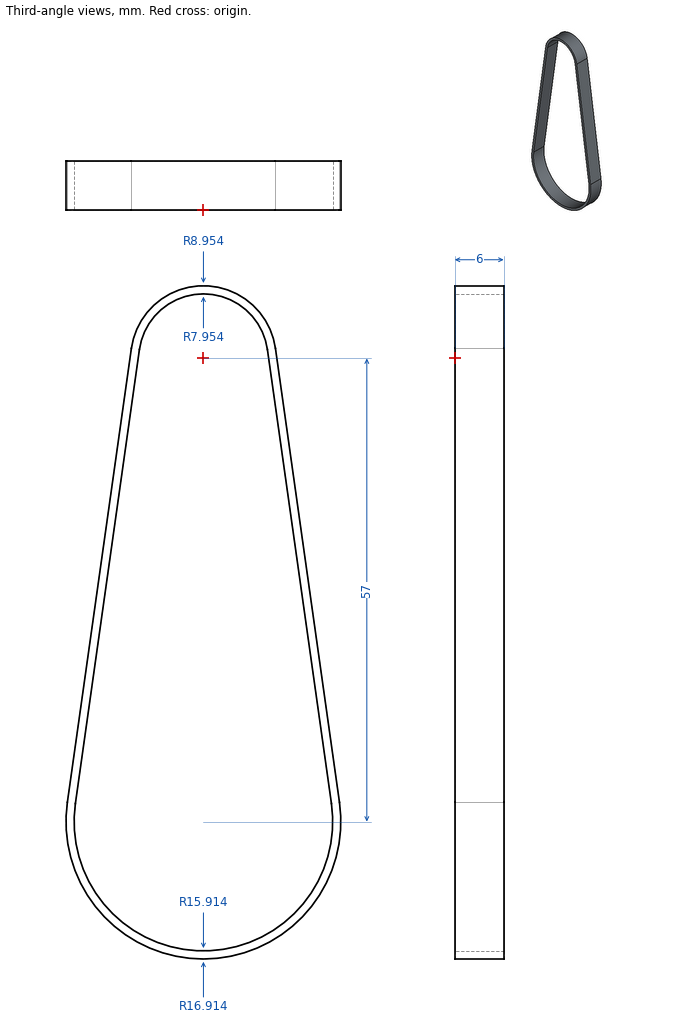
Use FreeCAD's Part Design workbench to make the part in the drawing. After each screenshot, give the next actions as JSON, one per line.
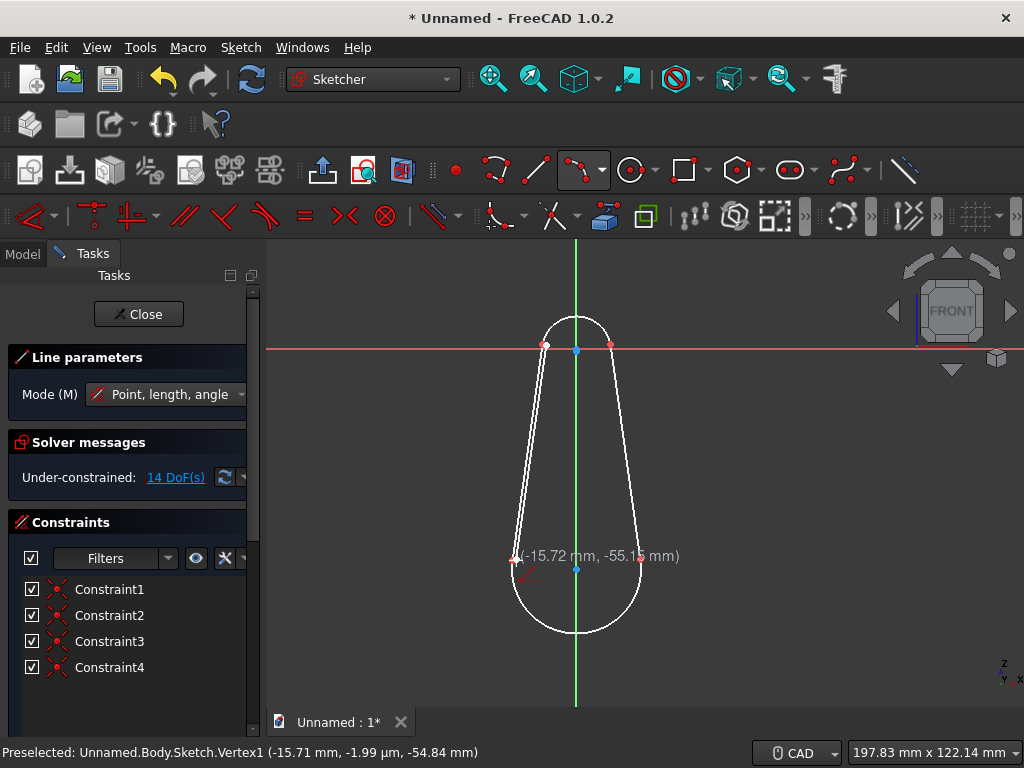
{"action": "scroll", "coordinate": [637, 559], "scroll_direction": "up", "scroll_amount": 8}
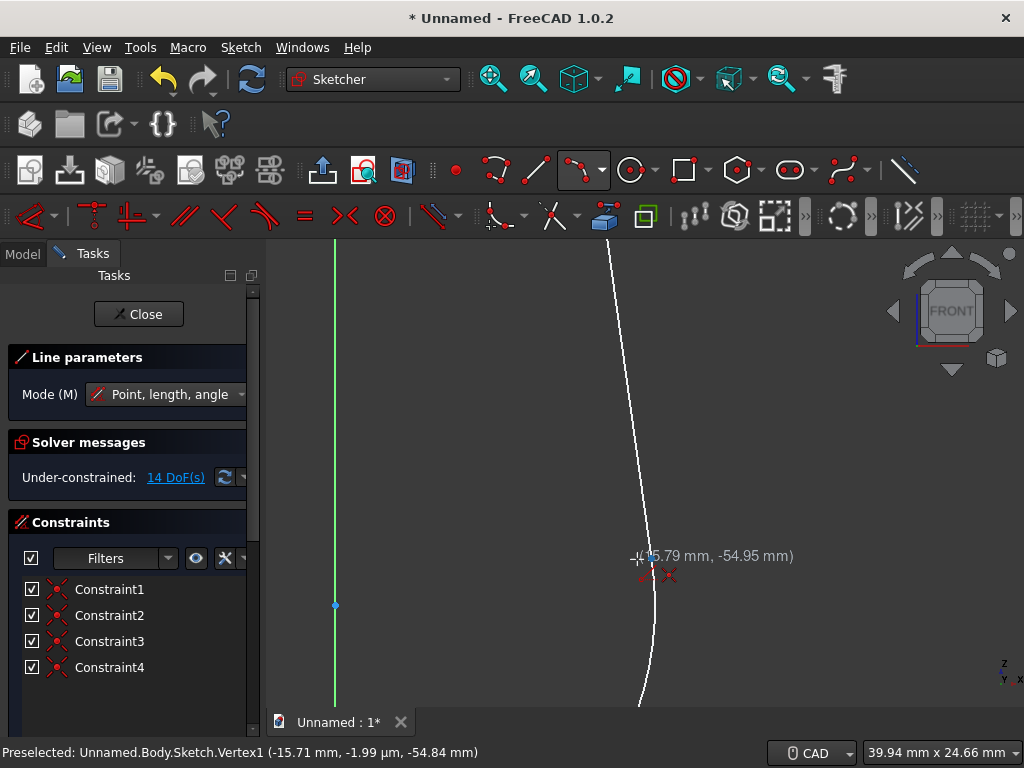
{"action": "left_click", "coordinate": [634, 558]}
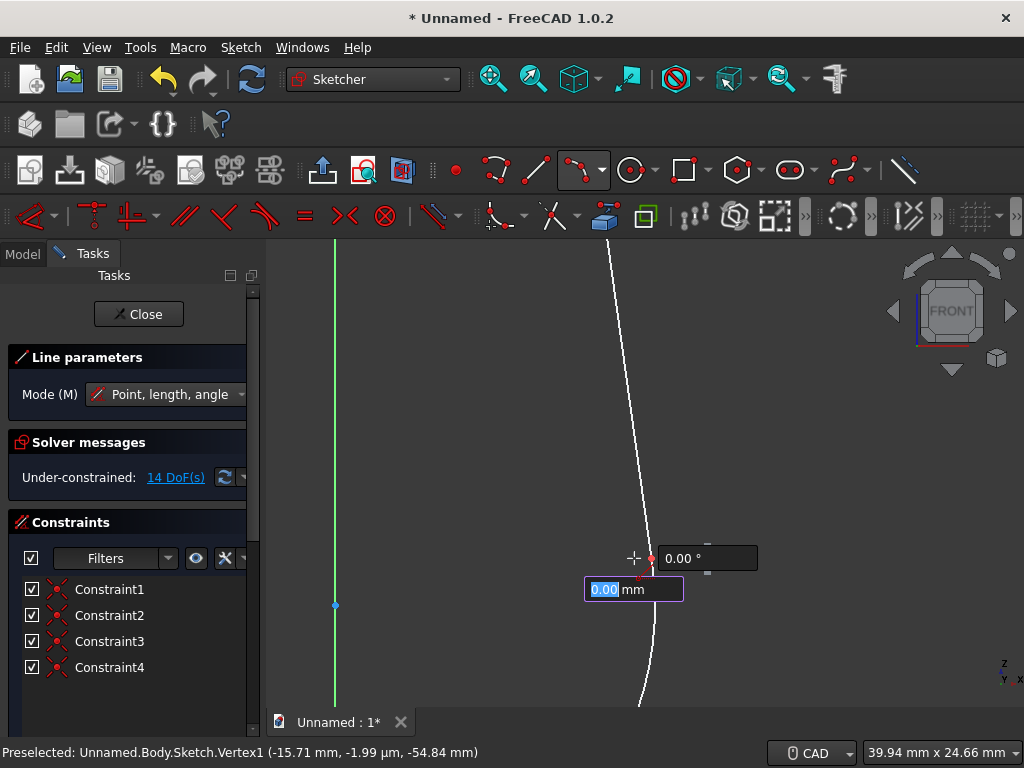
{"action": "scroll", "coordinate": [637, 559], "scroll_direction": "down", "scroll_amount": 8}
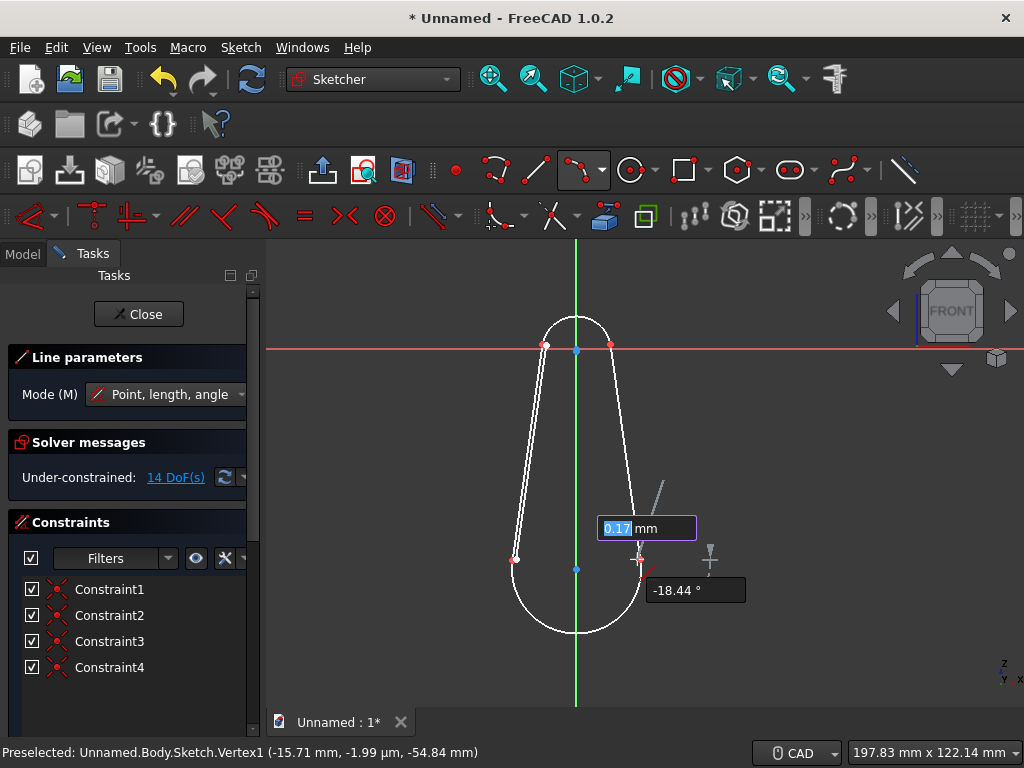
{"action": "scroll", "coordinate": [607, 345], "scroll_direction": "up", "scroll_amount": 8}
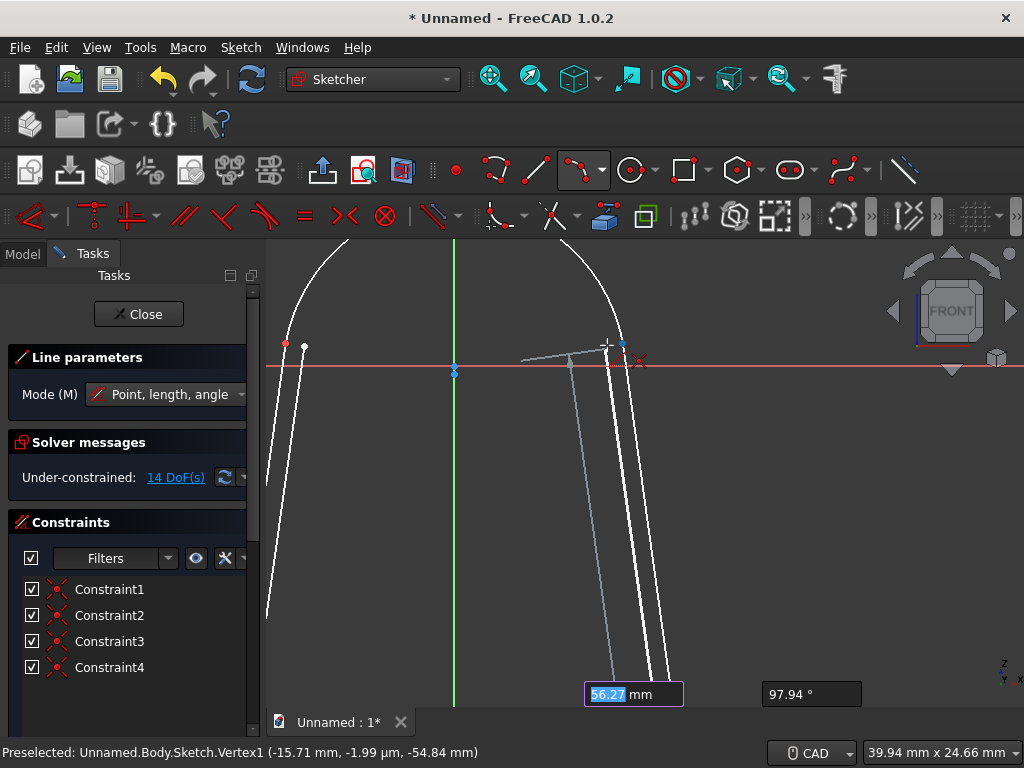
{"action": "left_click", "coordinate": [604, 345]}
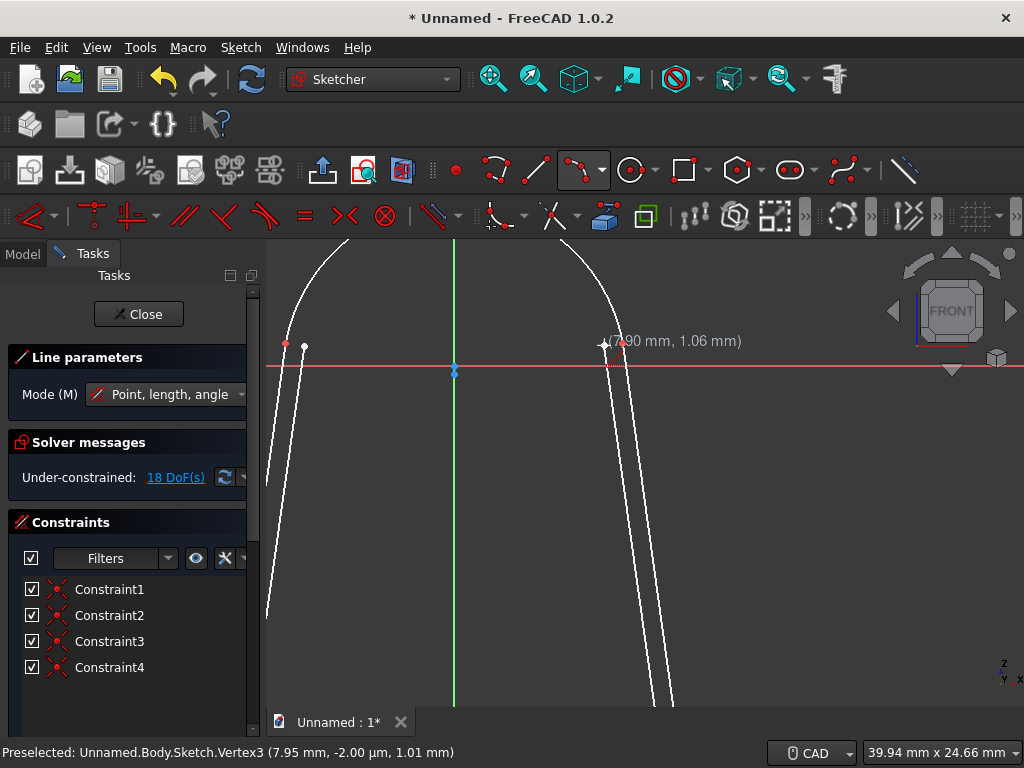
{"action": "left_click", "coordinate": [578, 170]}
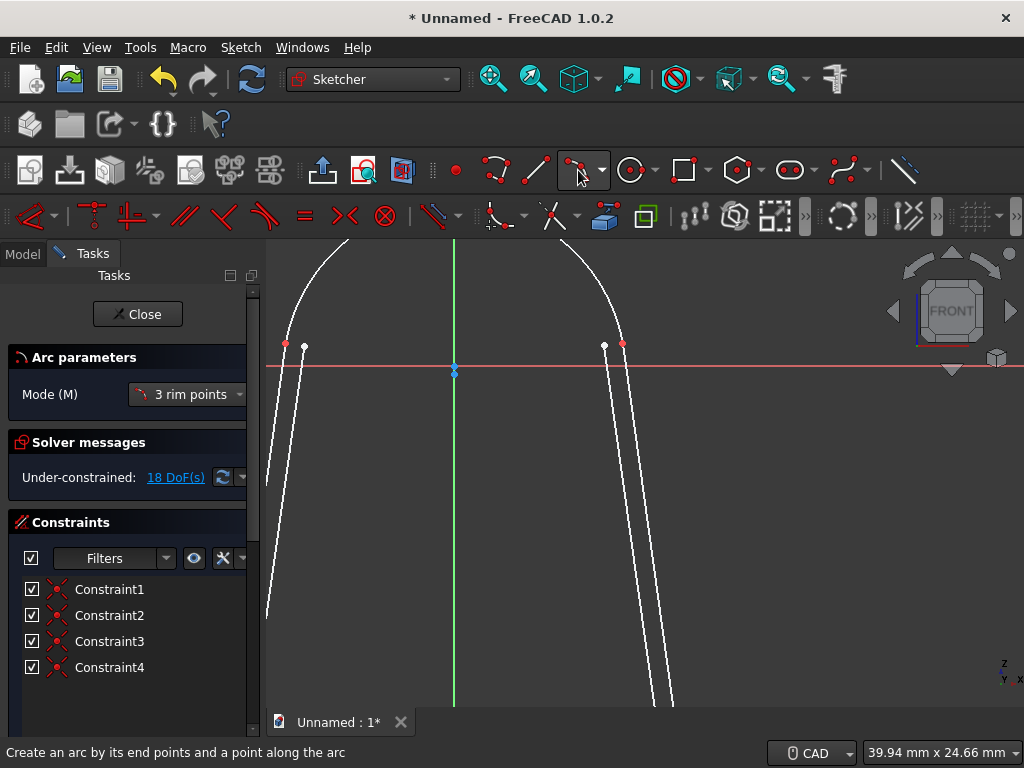
{"action": "scroll", "coordinate": [607, 344], "scroll_direction": "down", "scroll_amount": 8}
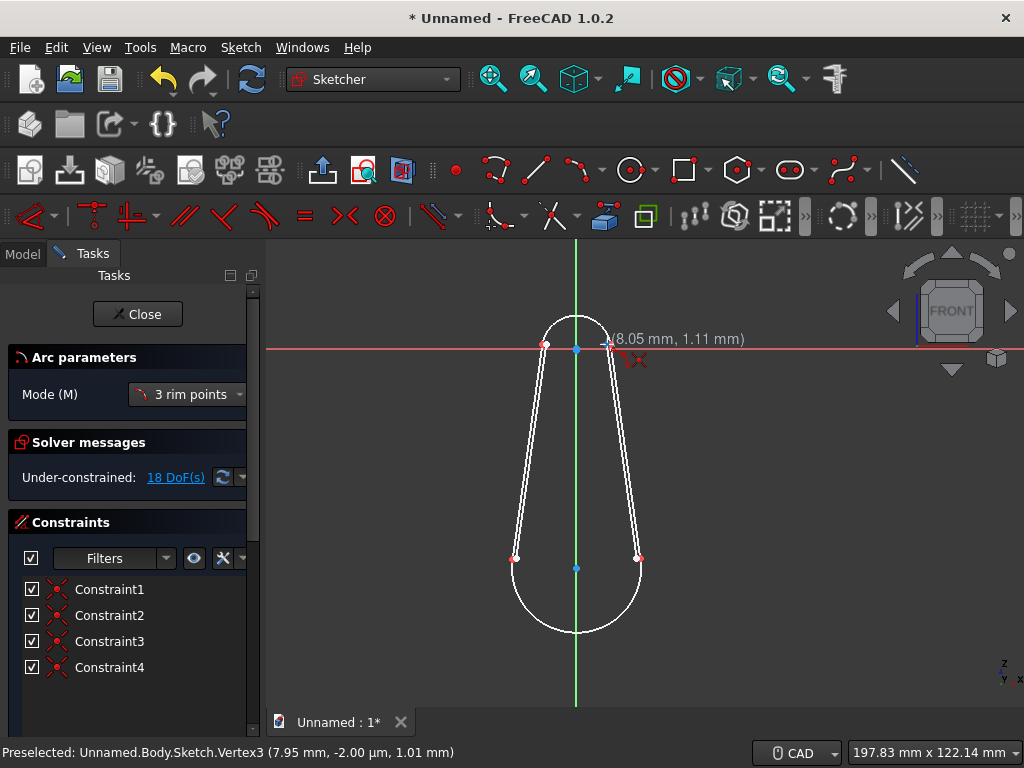
{"action": "scroll", "coordinate": [516, 559], "scroll_direction": "up", "scroll_amount": 8}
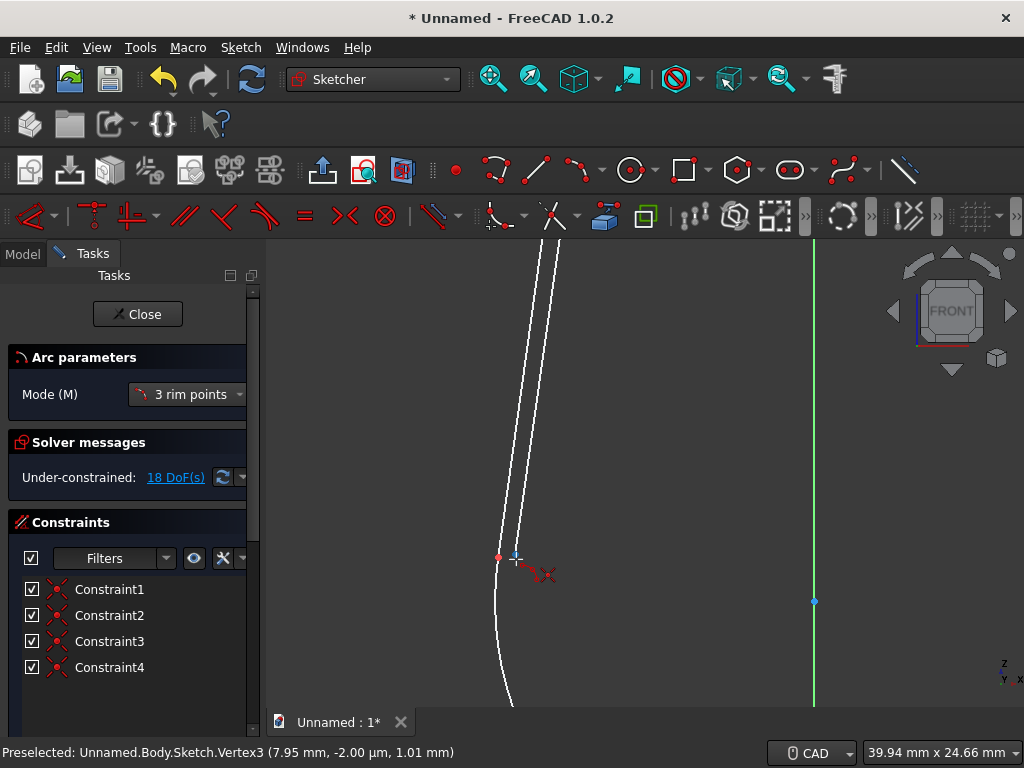
{"action": "left_click", "coordinate": [515, 555]}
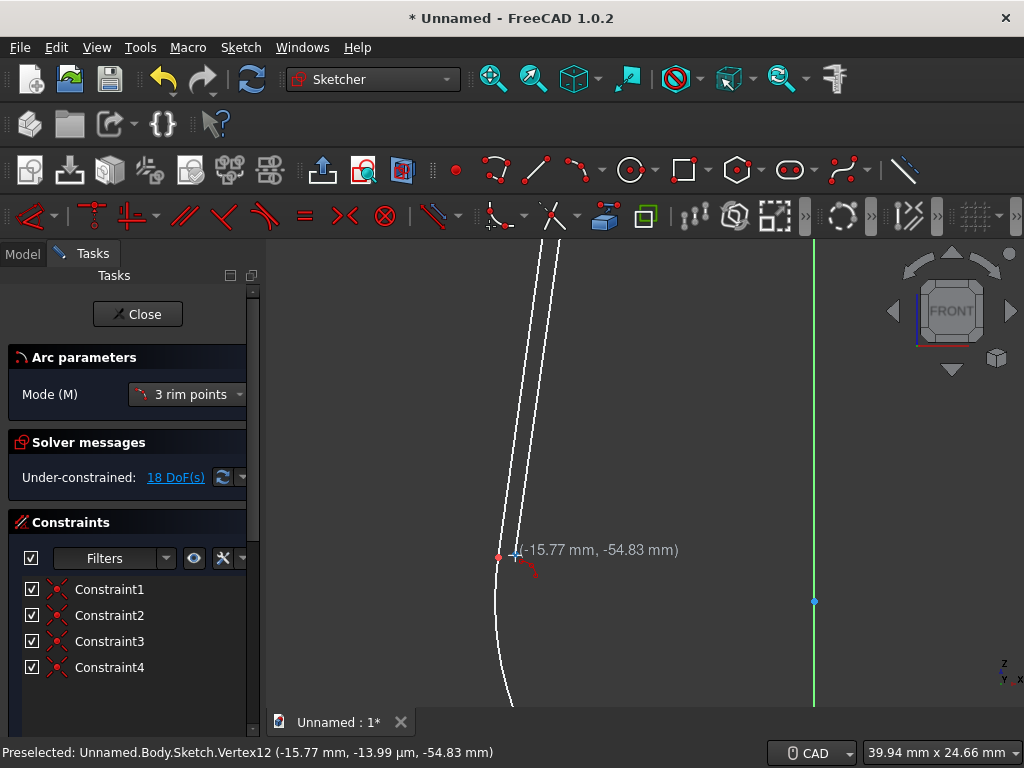
{"action": "scroll", "coordinate": [516, 560], "scroll_direction": "down", "scroll_amount": 8}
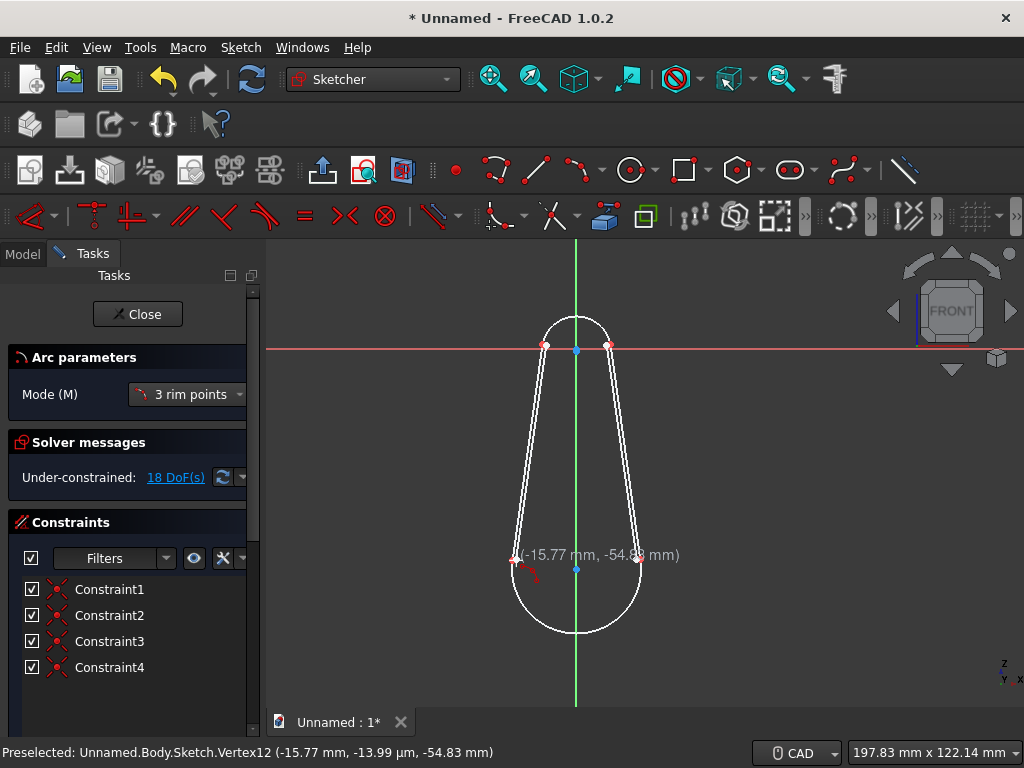
{"action": "scroll", "coordinate": [637, 559], "scroll_direction": "up", "scroll_amount": 8}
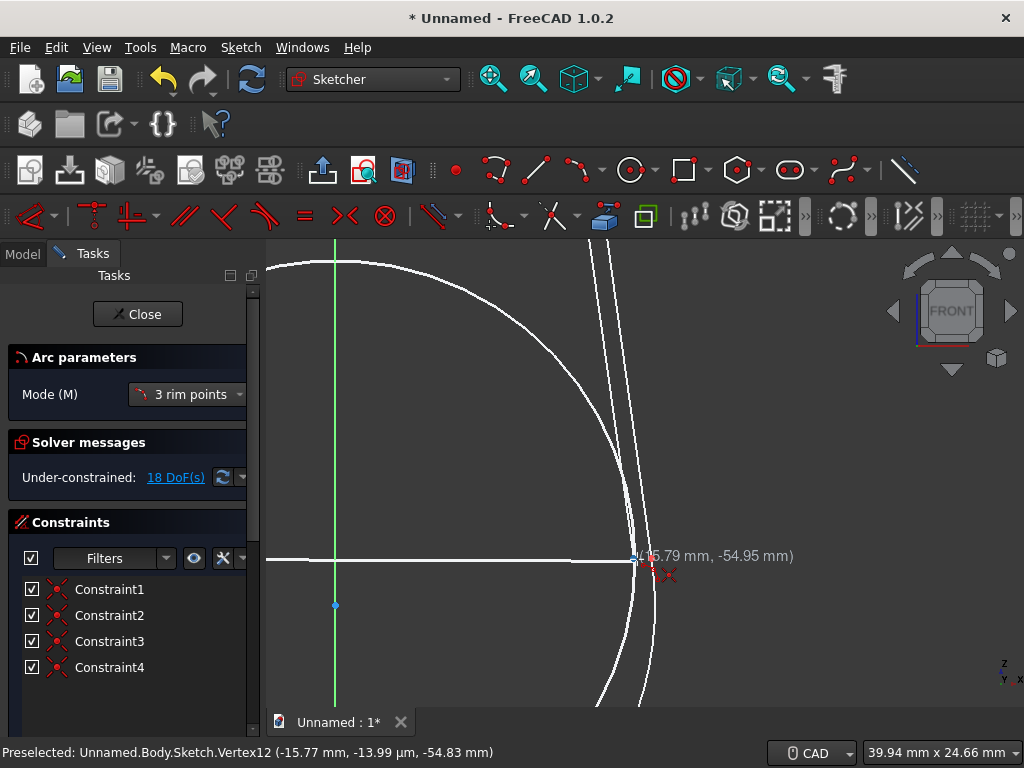
{"action": "left_click", "coordinate": [634, 559]}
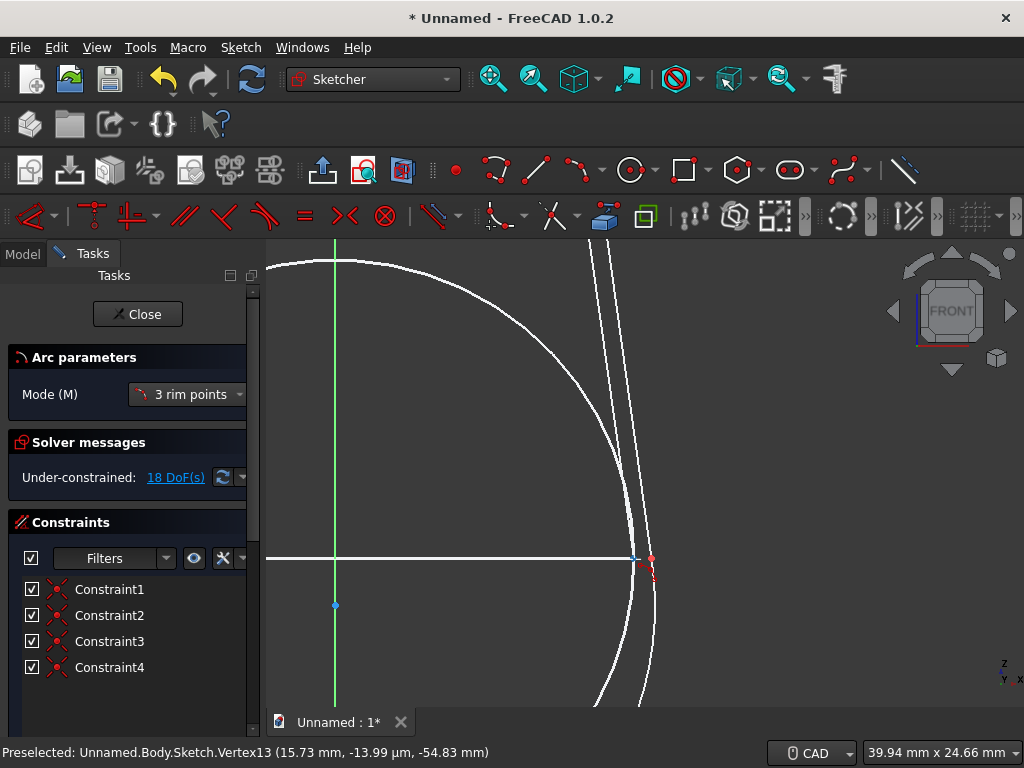
{"action": "scroll", "coordinate": [637, 559], "scroll_direction": "down", "scroll_amount": 8}